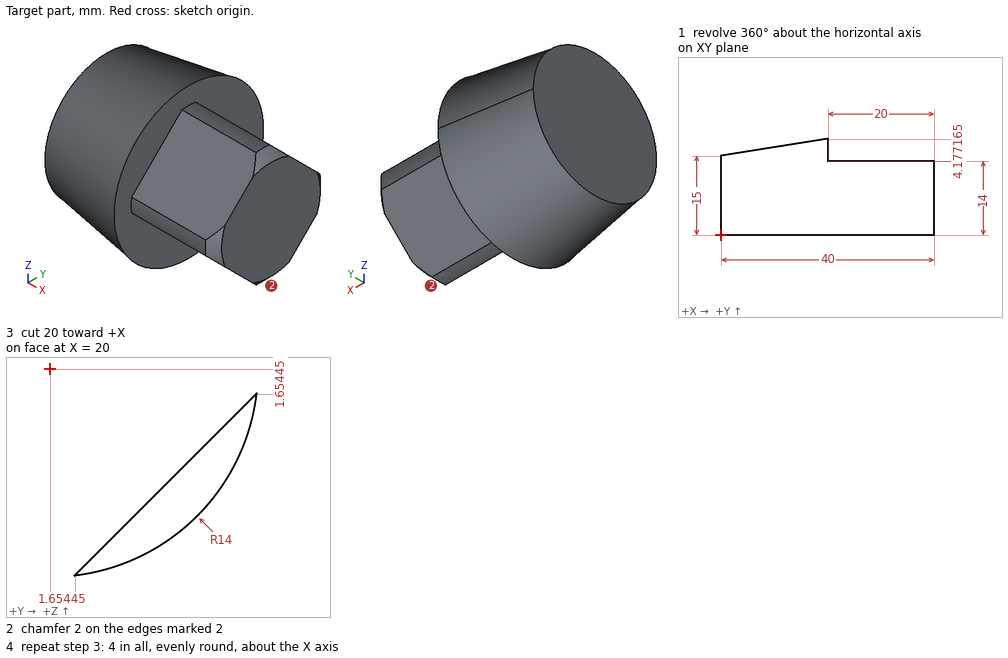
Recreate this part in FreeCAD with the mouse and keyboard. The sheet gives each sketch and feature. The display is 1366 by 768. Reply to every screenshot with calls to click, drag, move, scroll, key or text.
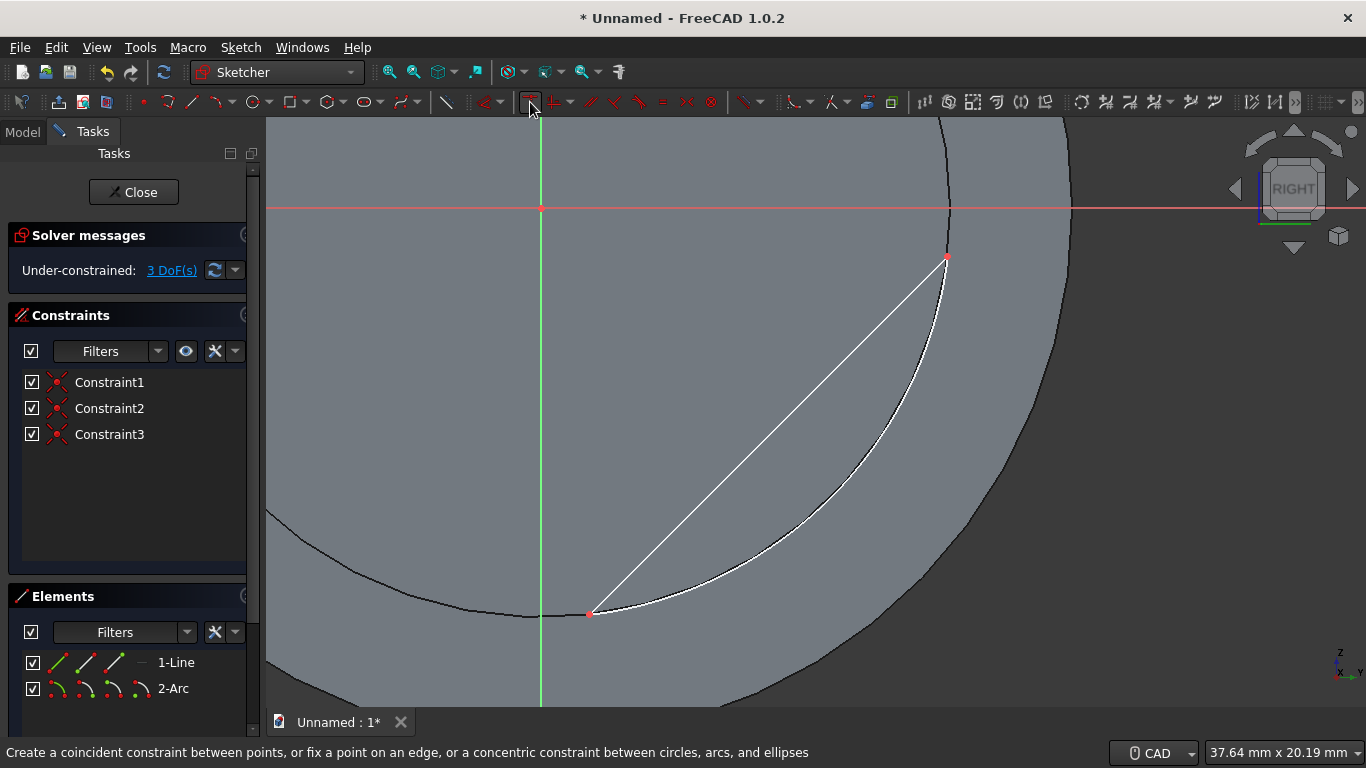
click(744, 564)
click(760, 592)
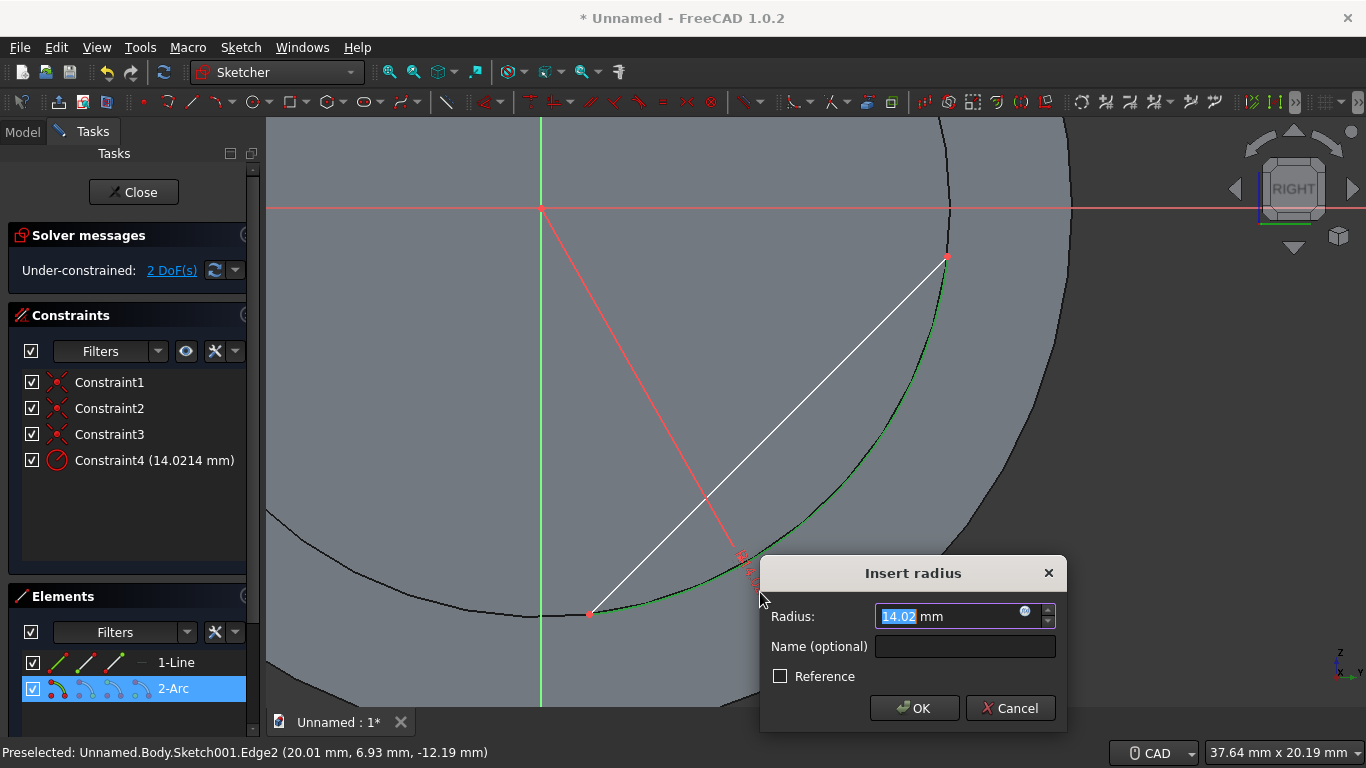
text(14)
key(Return)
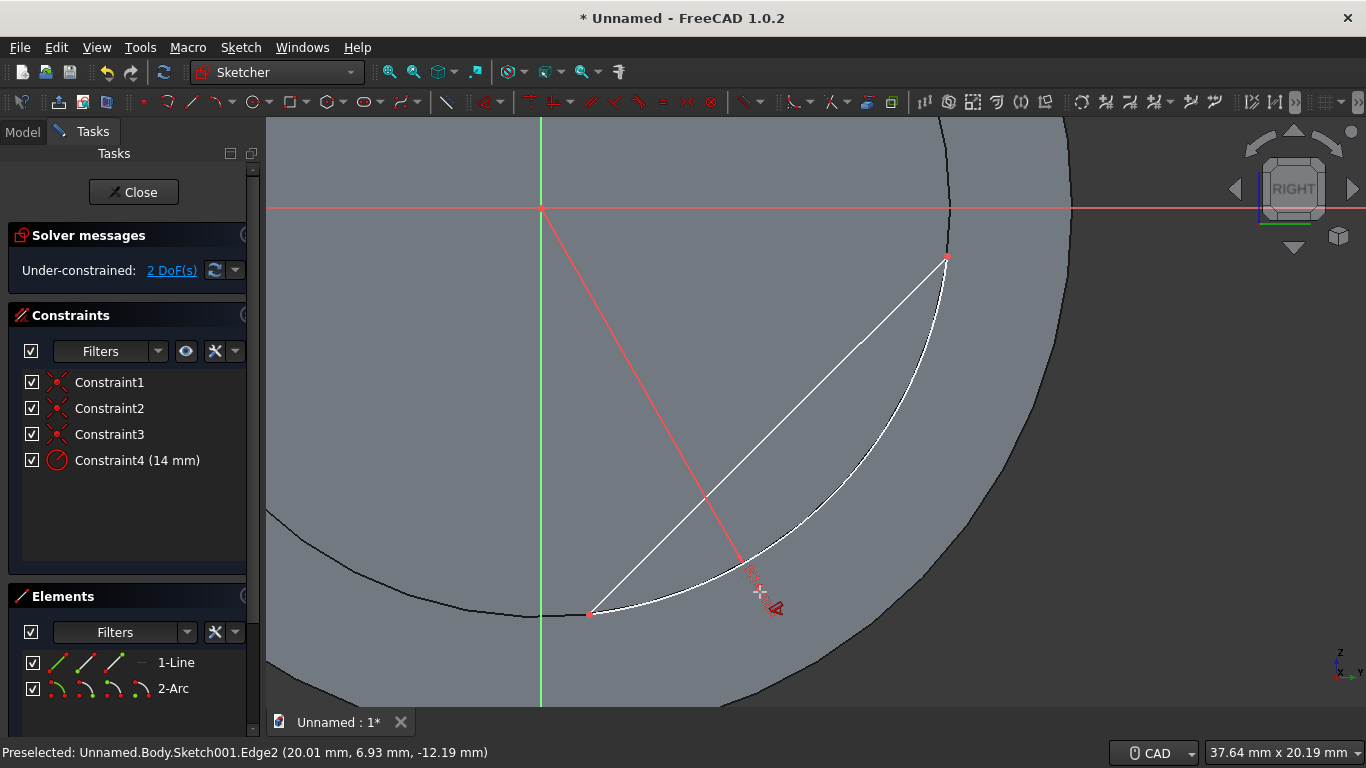
click(947, 257)
click(507, 233)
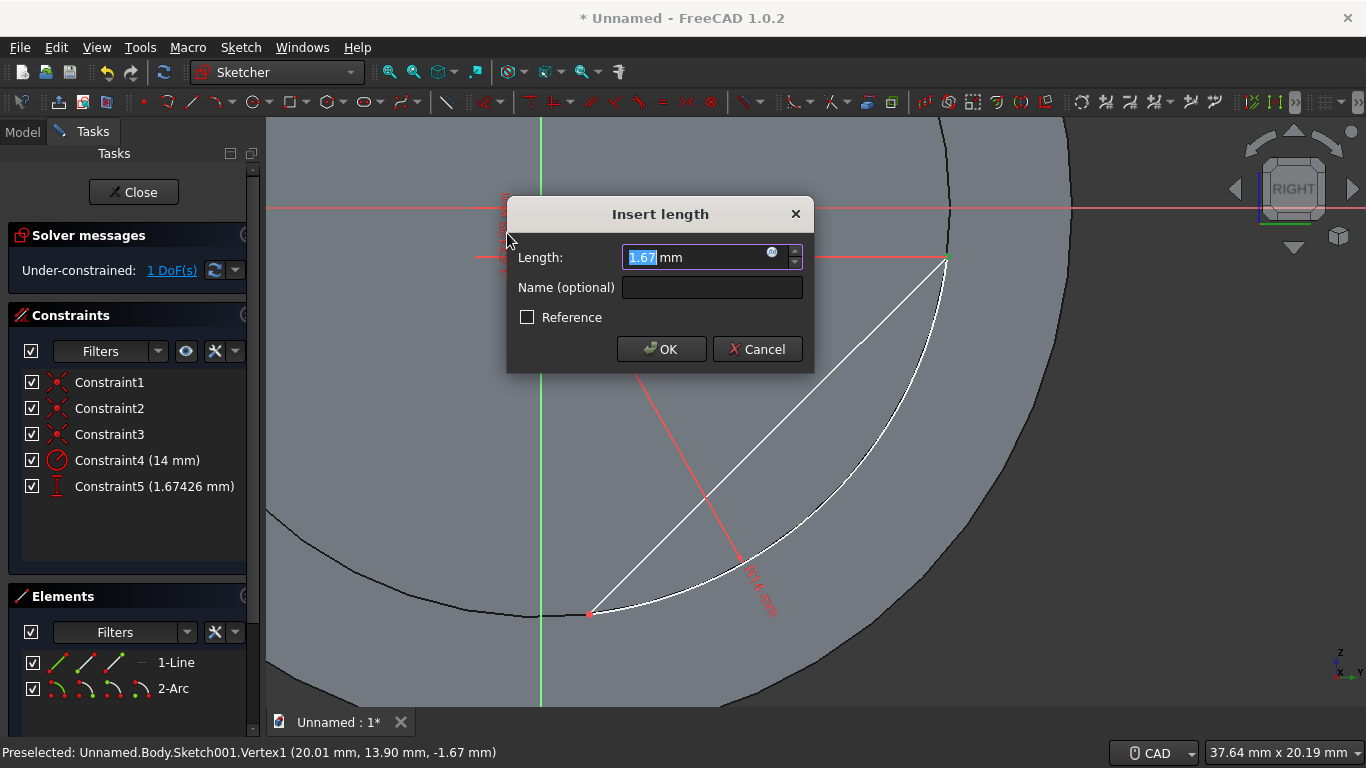
text(1.65445)
key(Return)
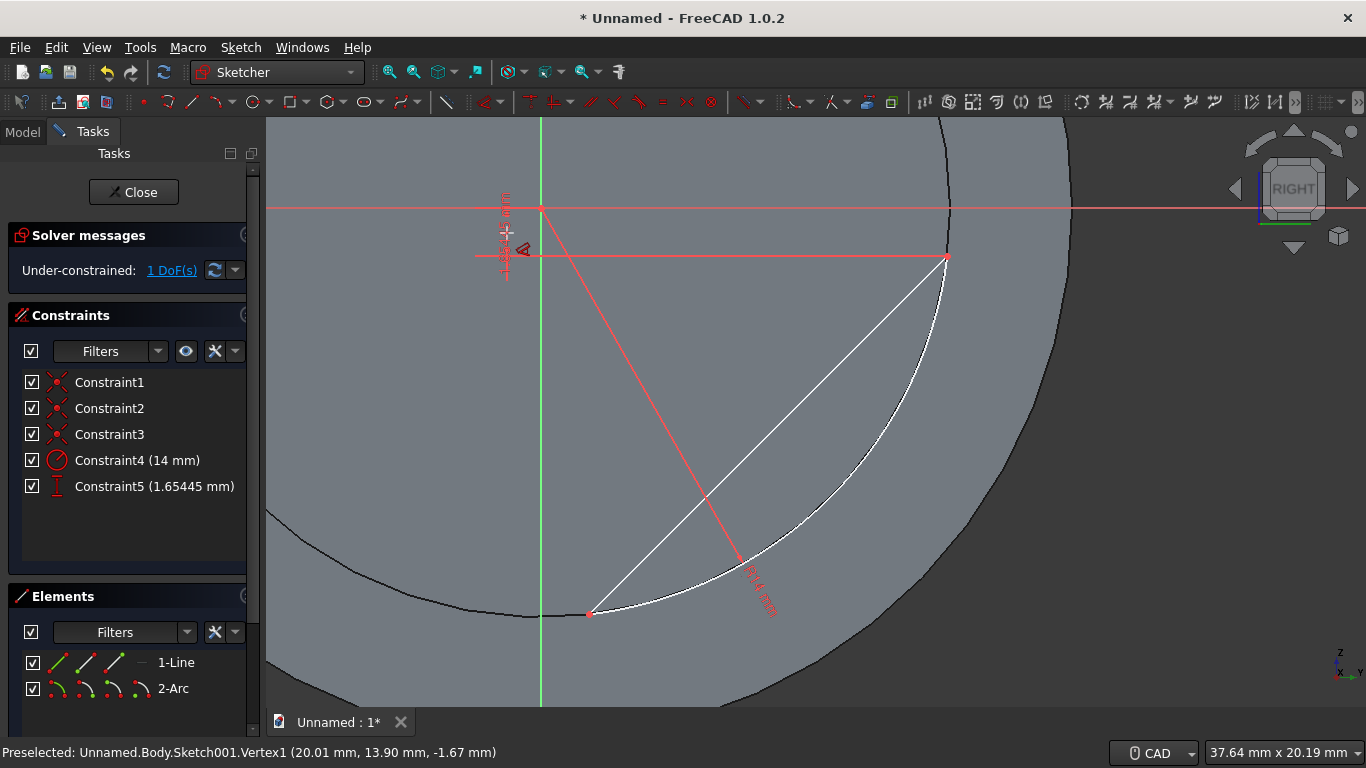
click(589, 614)
click(565, 648)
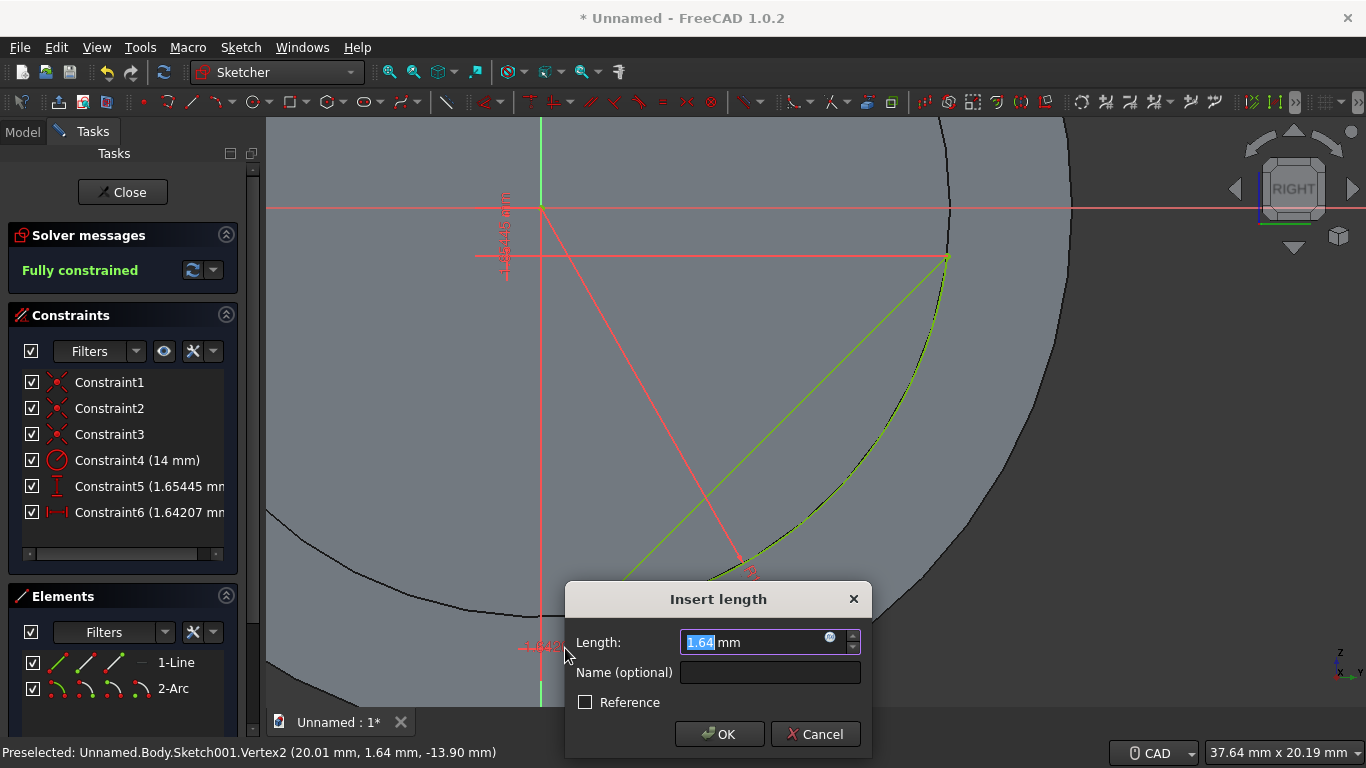
text(1.65445)
key(Return)
key(Escape)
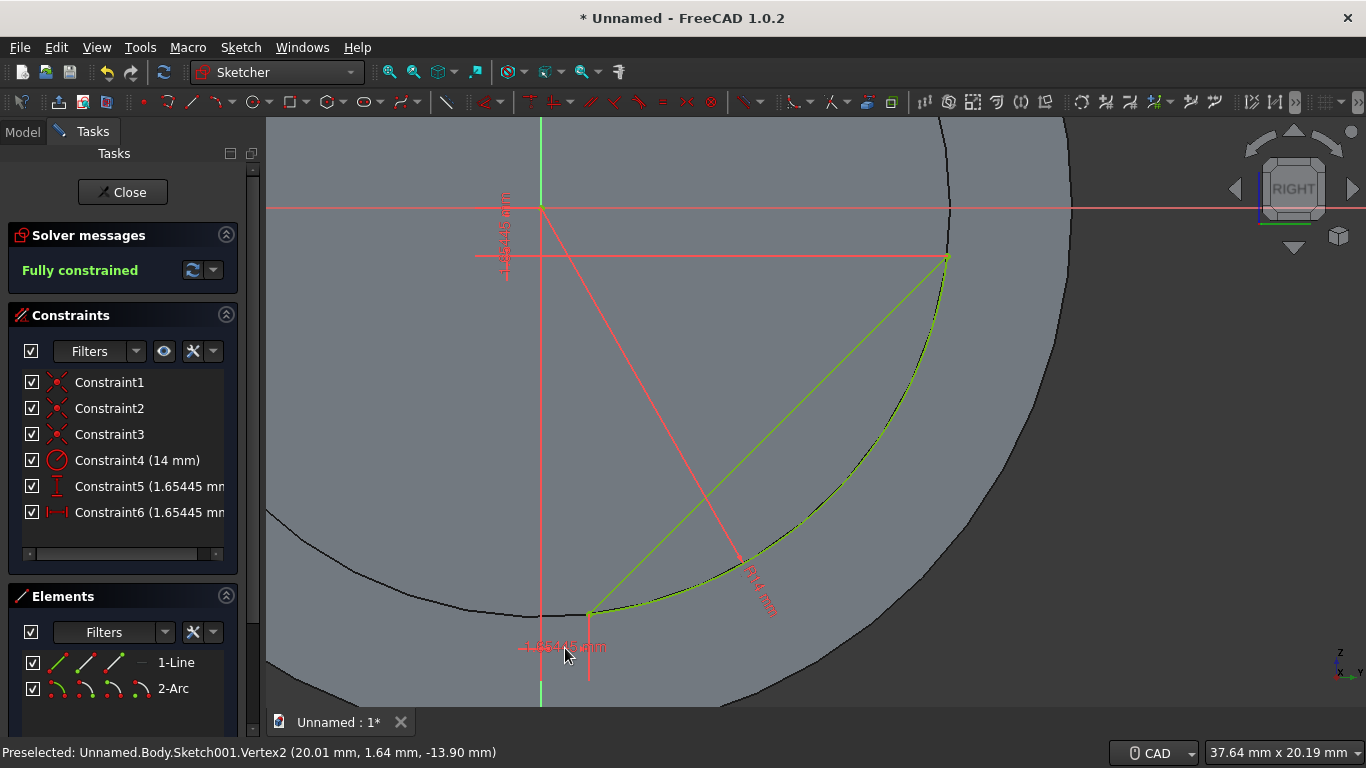
click(123, 192)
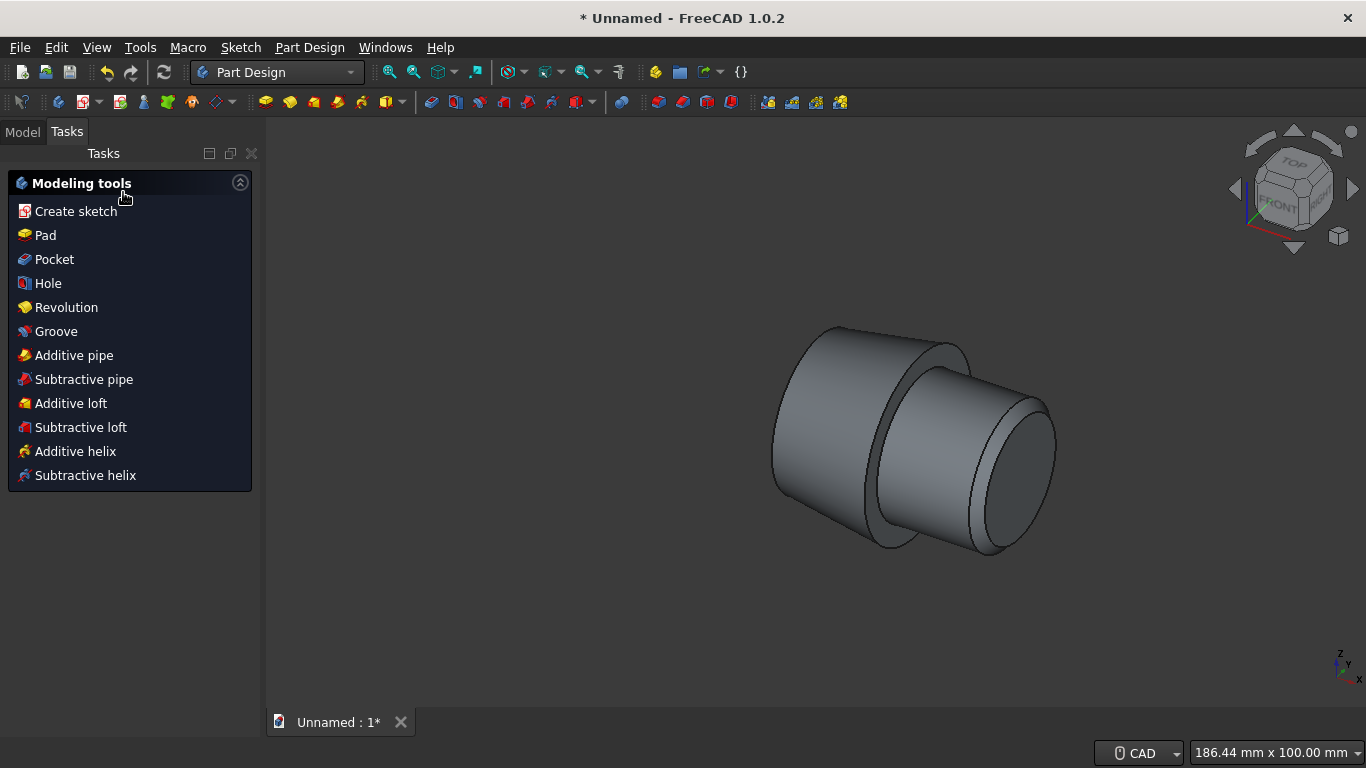
click(432, 102)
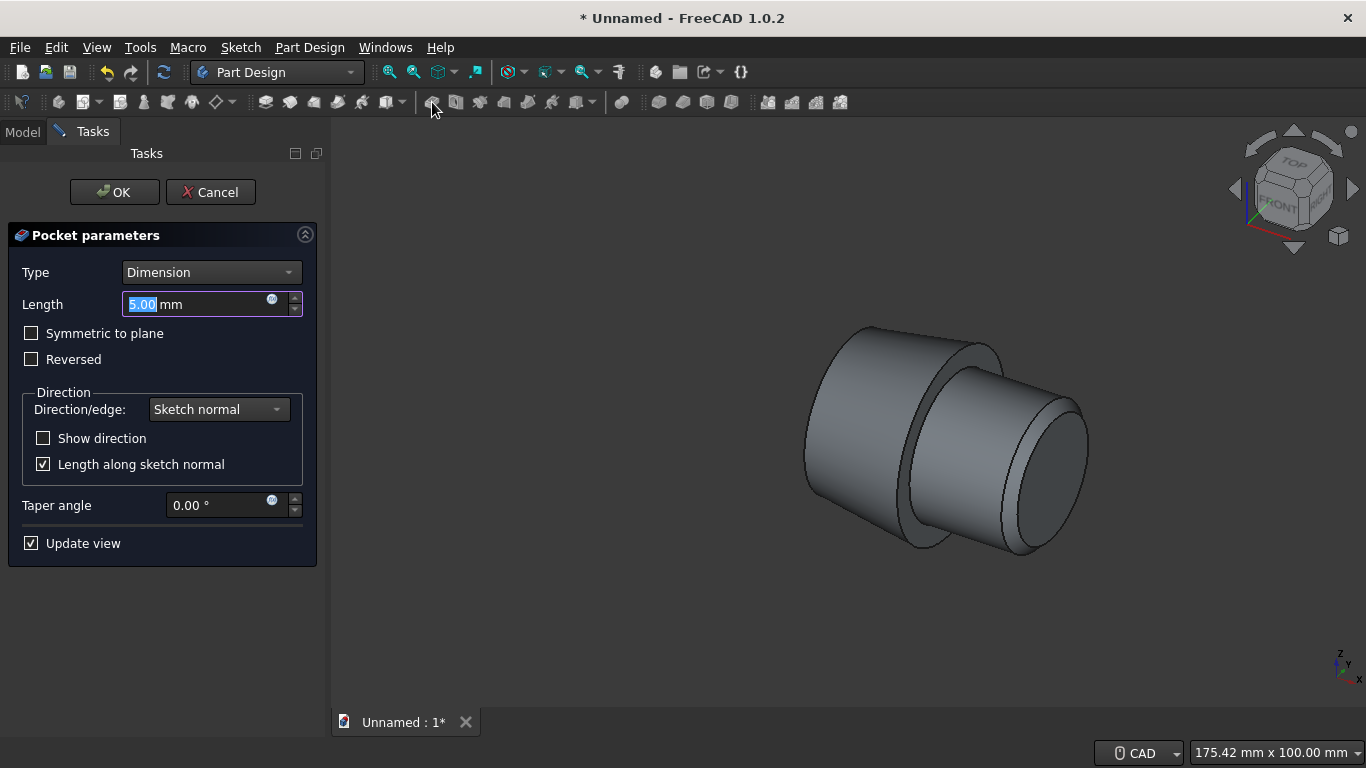
text(20)
key(Tab)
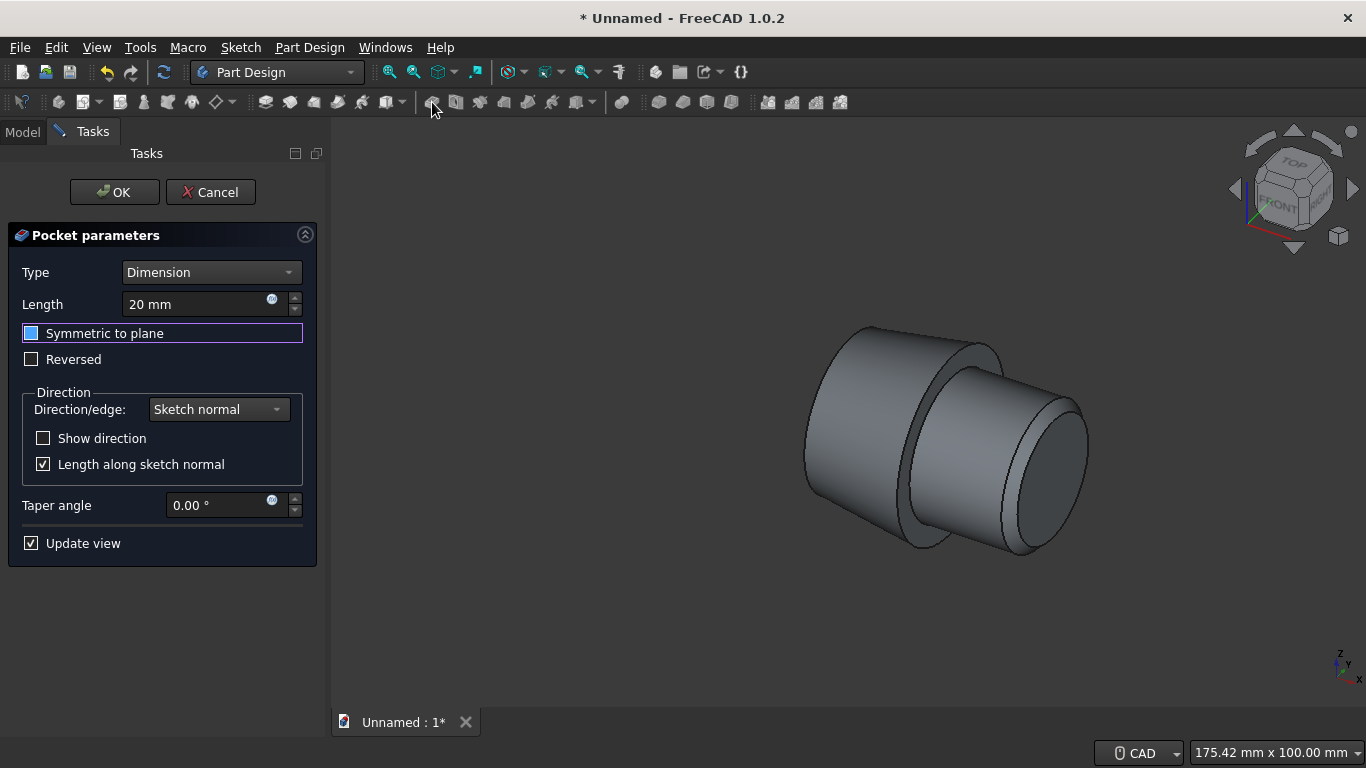
click(30, 359)